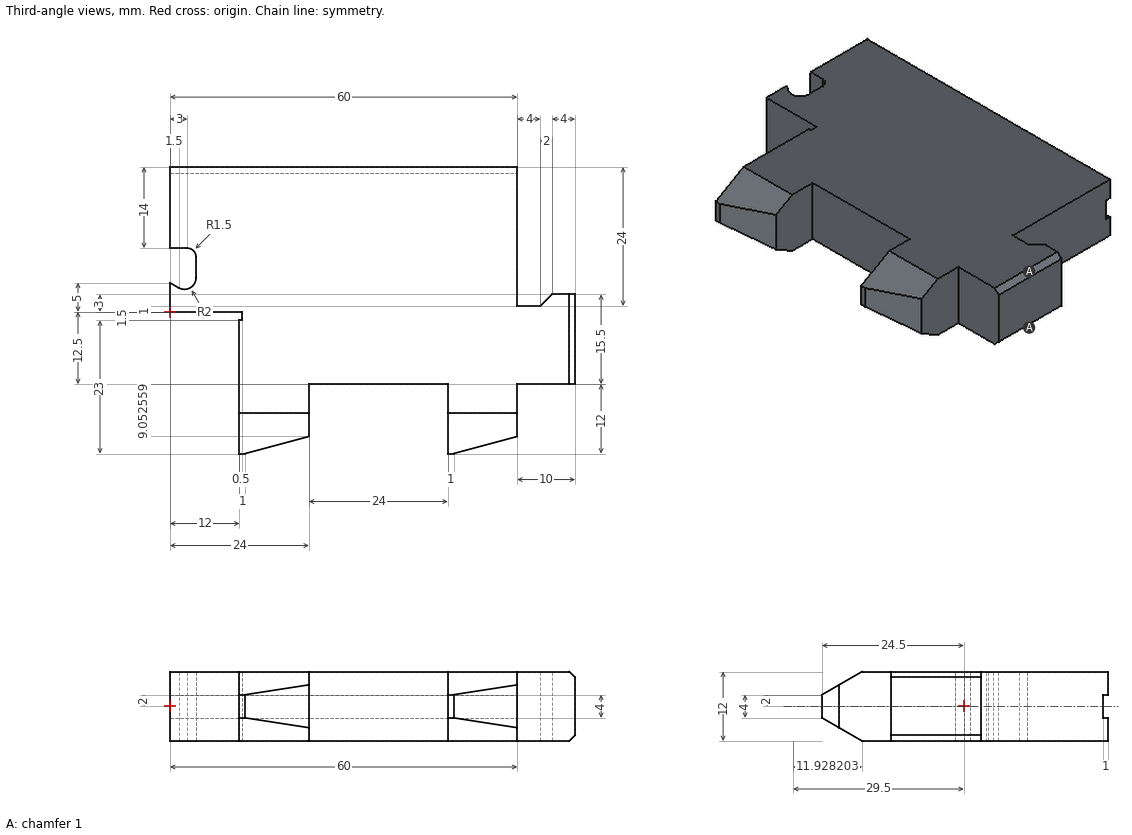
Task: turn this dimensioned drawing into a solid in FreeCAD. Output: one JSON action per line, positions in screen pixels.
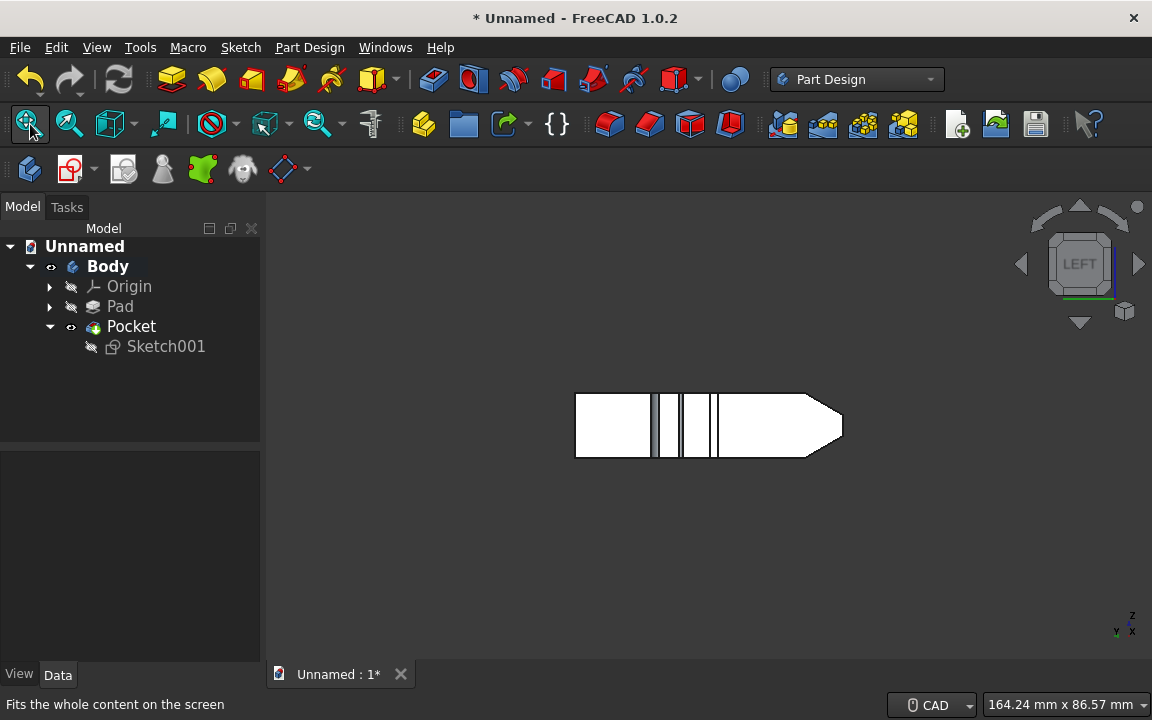
{"action": "key", "text": "4"}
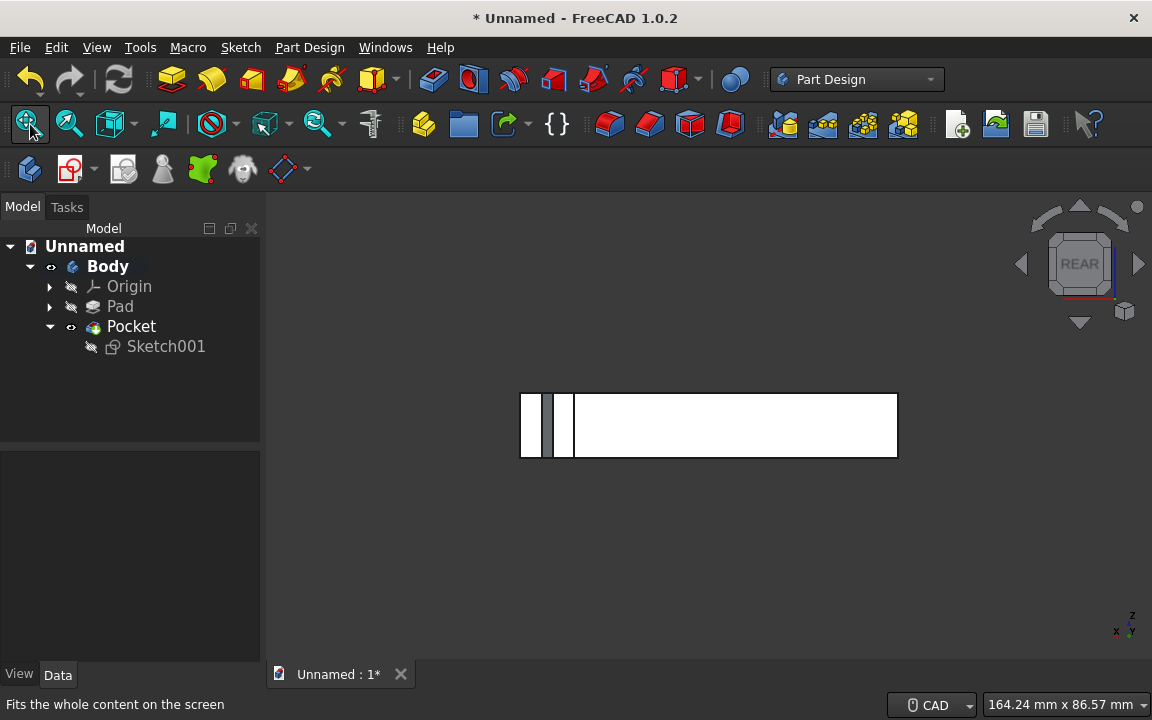
{"action": "left_click", "coordinate": [30, 124]}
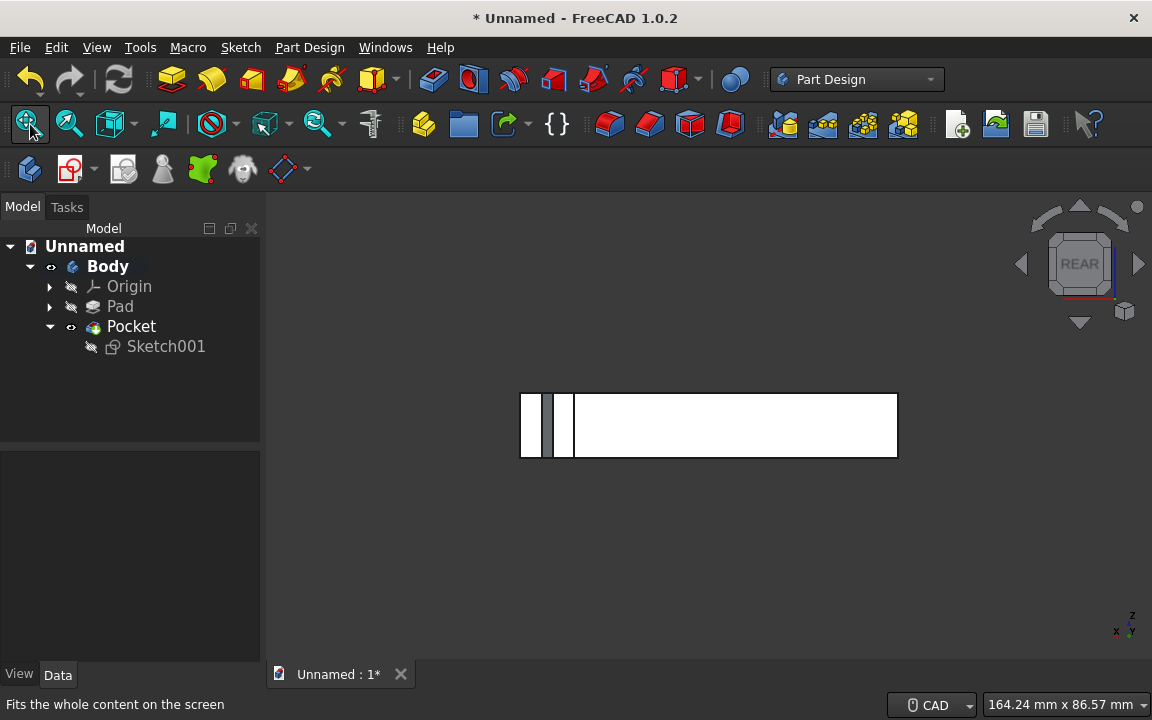
{"action": "left_click", "coordinate": [643, 425]}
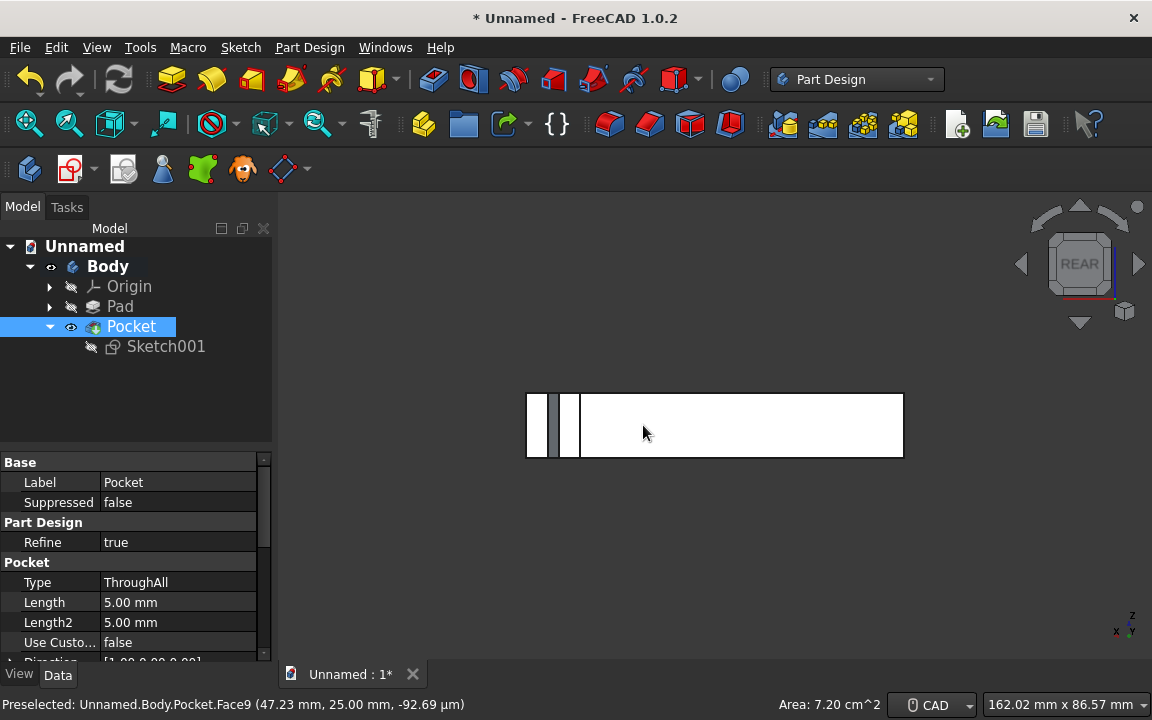
{"action": "left_click", "coordinate": [70, 170]}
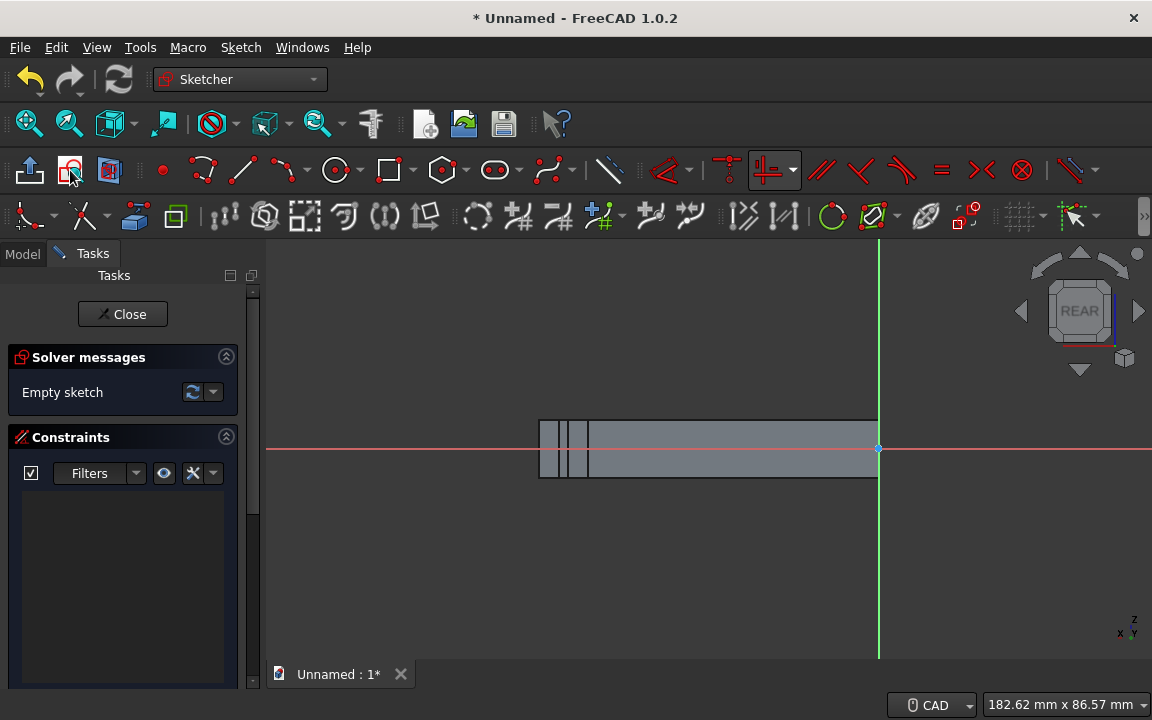
{"action": "scroll", "coordinate": [846, 449], "scroll_direction": "up", "scroll_amount": 3}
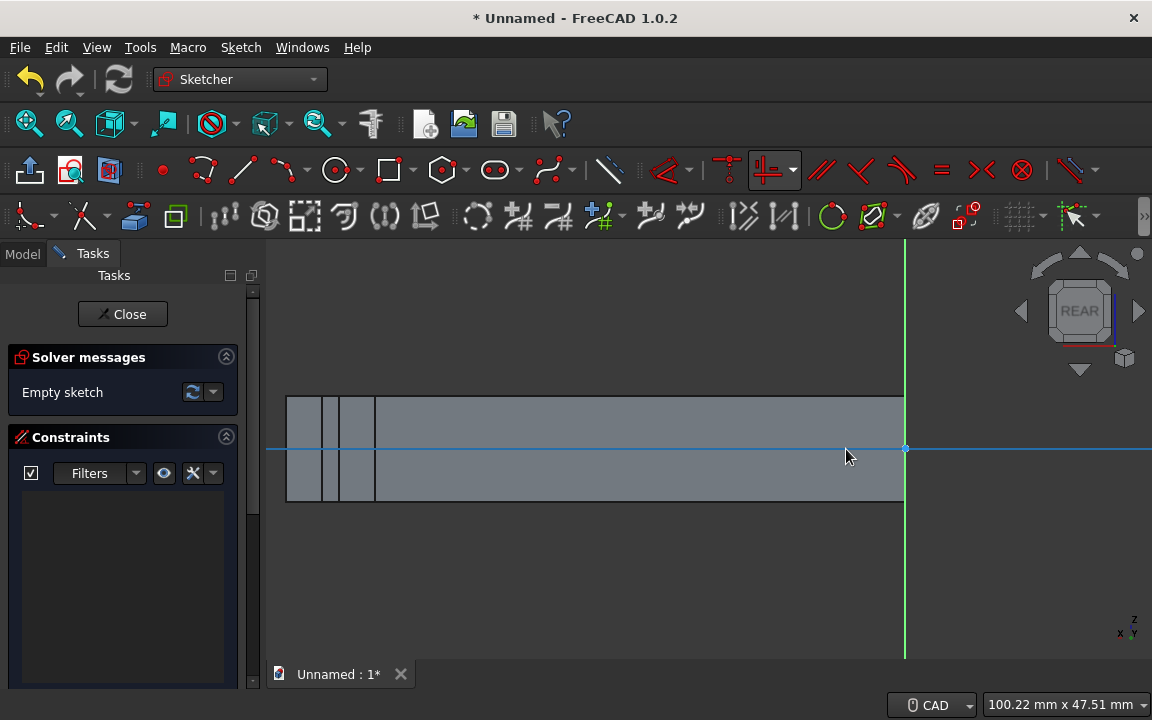
{"action": "left_click", "coordinate": [390, 170]}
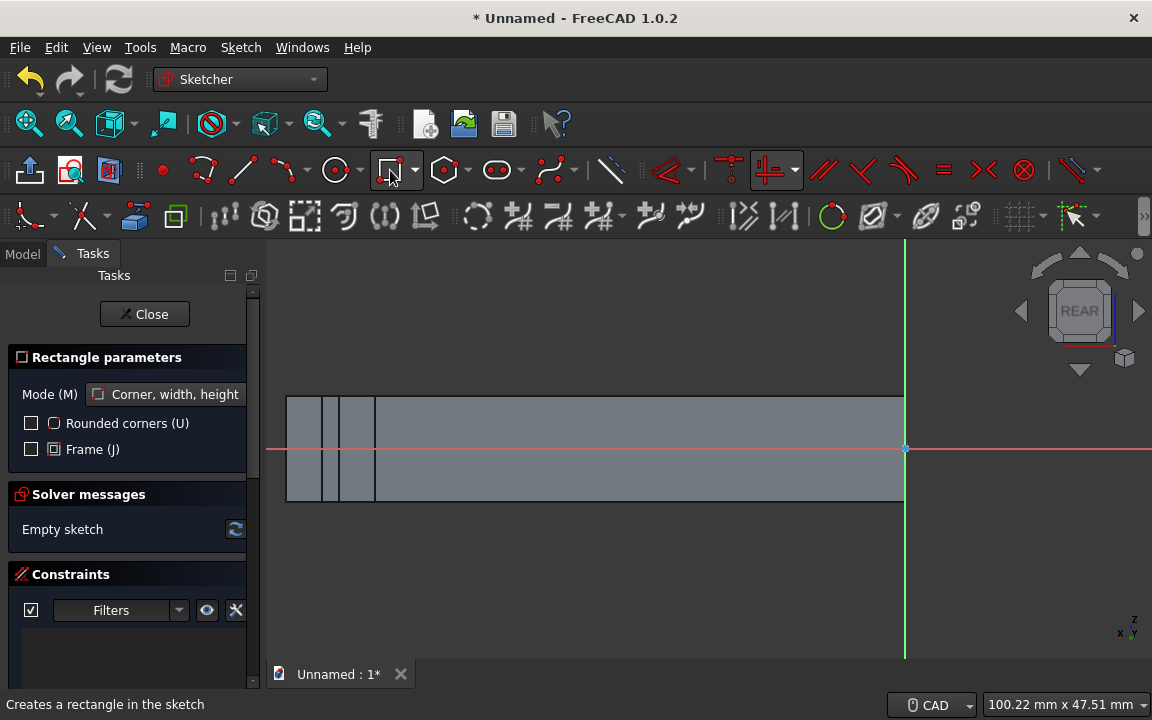
{"action": "left_click", "coordinate": [375, 431]}
{"action": "left_click", "coordinate": [905, 466]}
{"action": "key", "text": "Escape"}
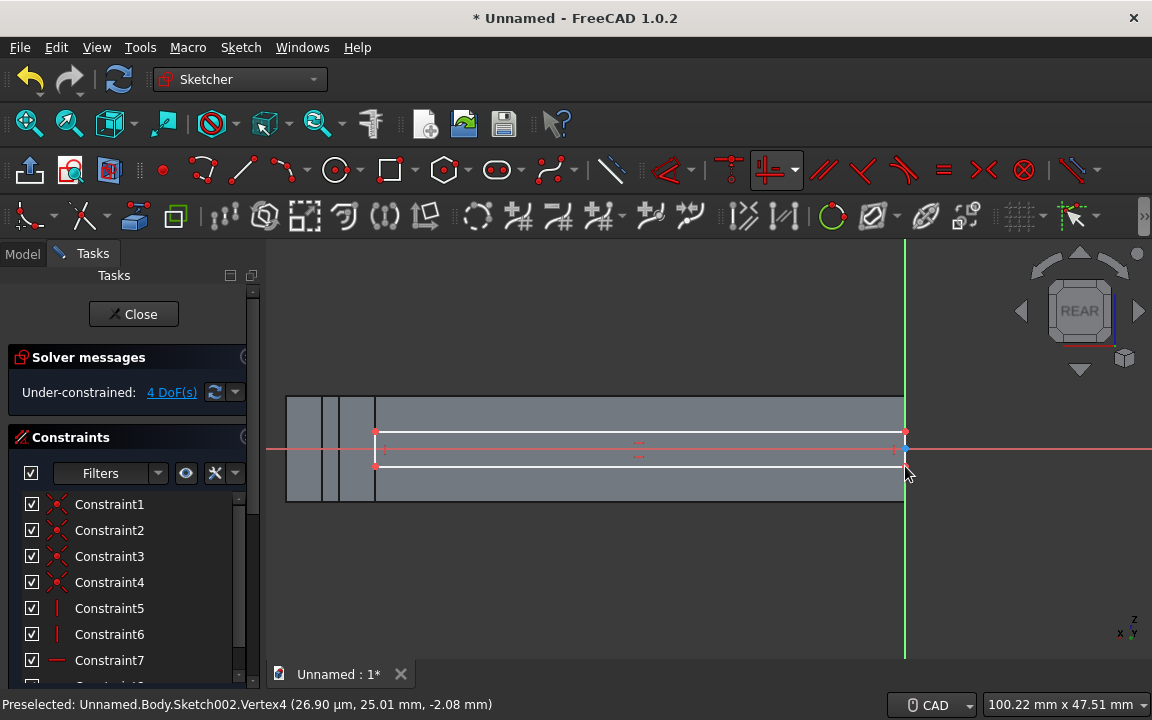
{"action": "left_click", "coordinate": [905, 467]}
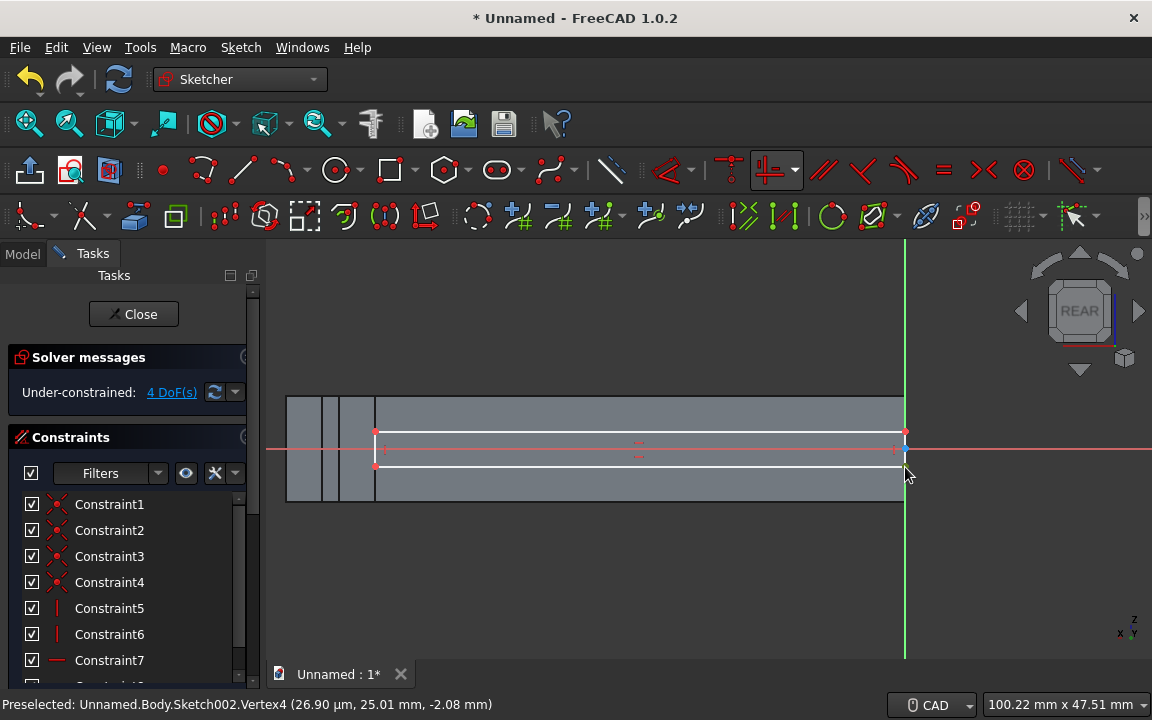
{"action": "left_click", "coordinate": [905, 605]}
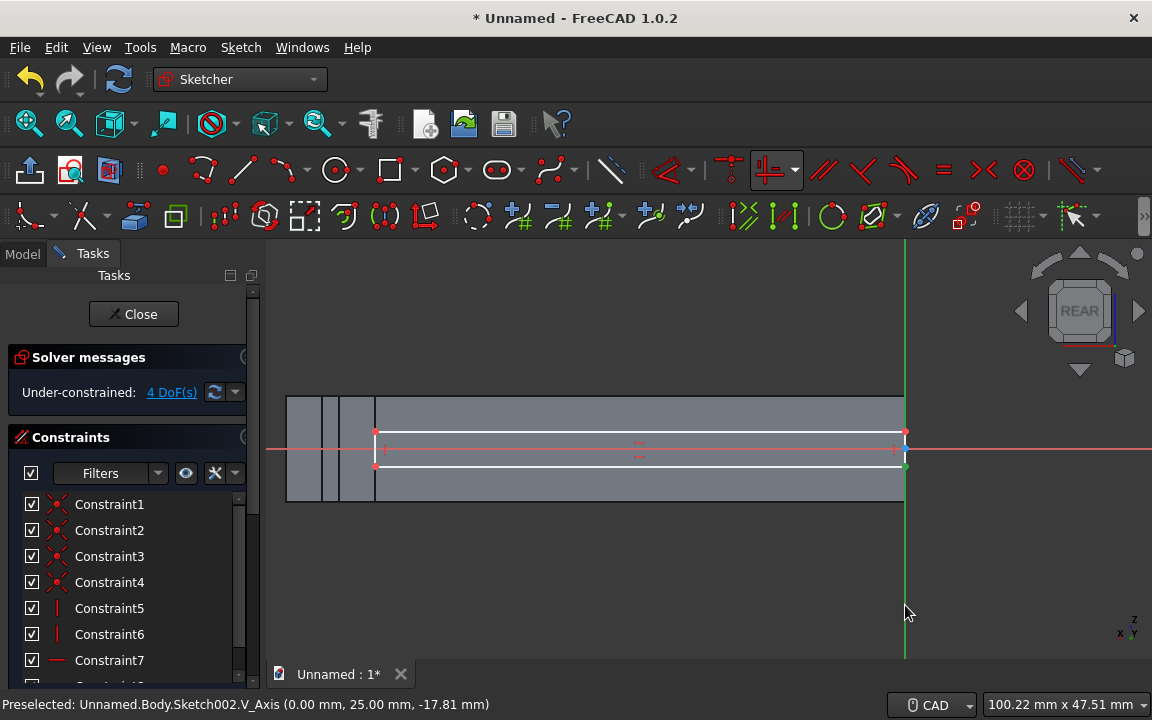
{"action": "left_click", "coordinate": [730, 170]}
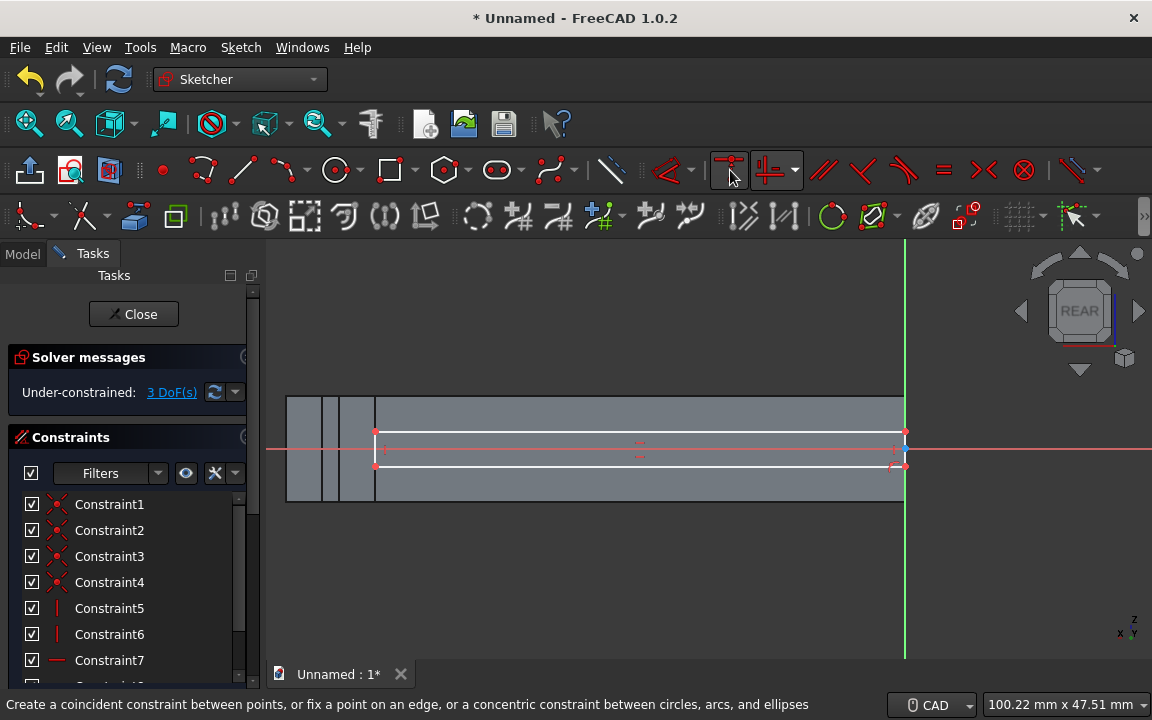
{"action": "left_click", "coordinate": [666, 170]}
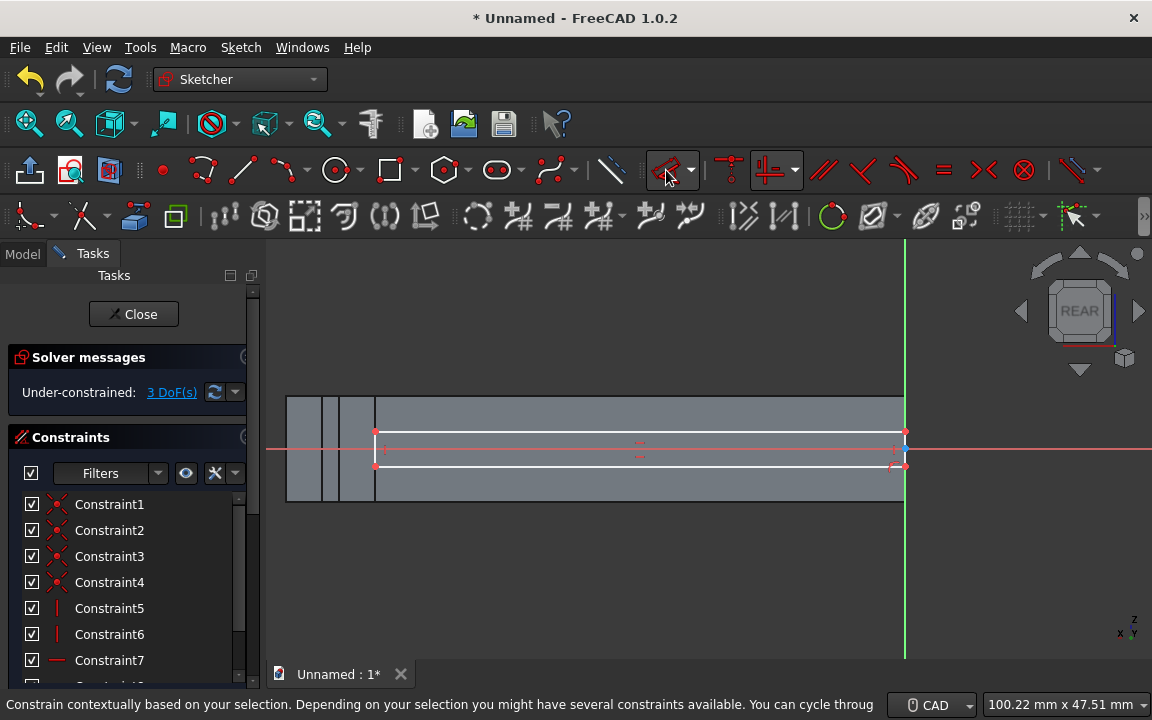
{"action": "left_click", "coordinate": [375, 446]}
{"action": "left_click", "coordinate": [341, 462]}